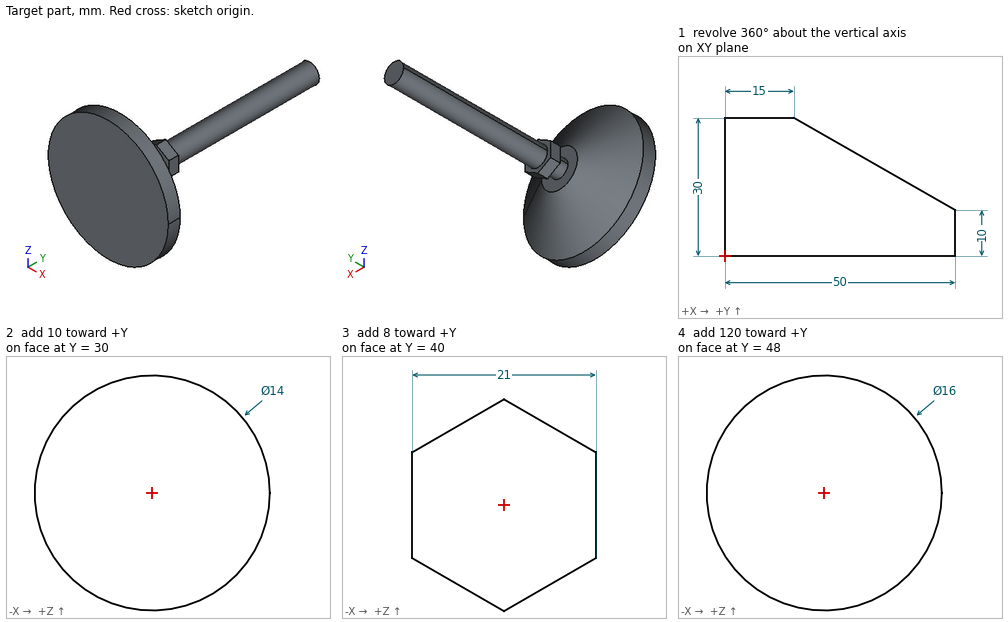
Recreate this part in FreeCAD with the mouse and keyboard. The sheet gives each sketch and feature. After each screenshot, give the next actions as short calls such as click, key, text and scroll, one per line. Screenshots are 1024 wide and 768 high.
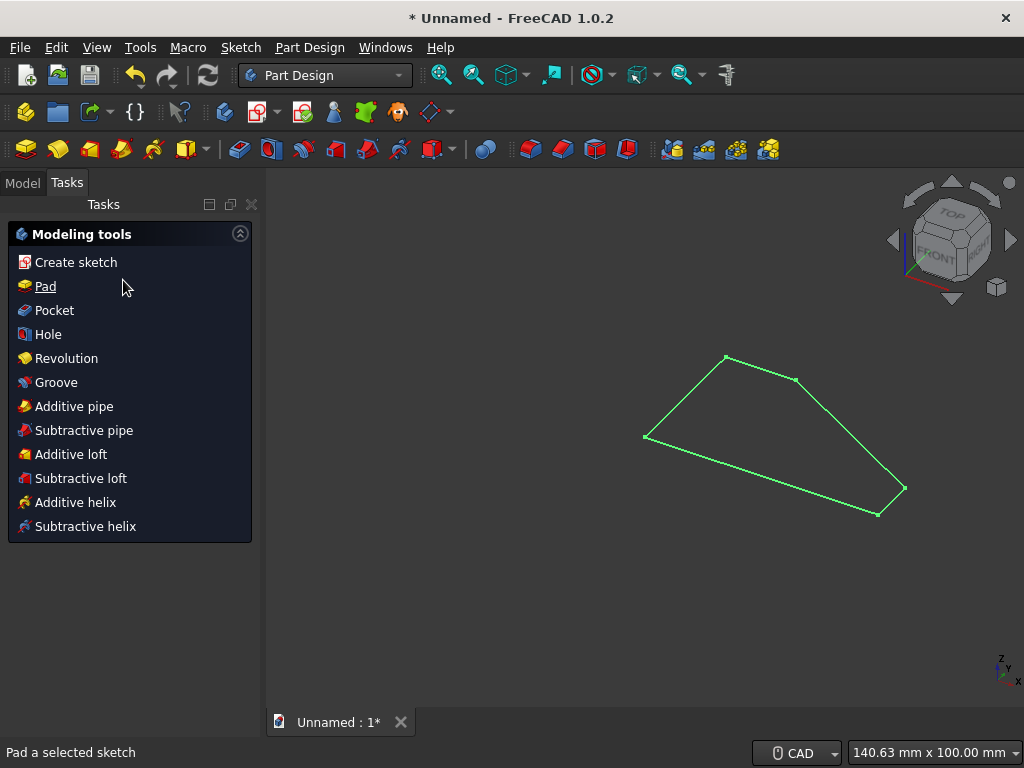
click(58, 150)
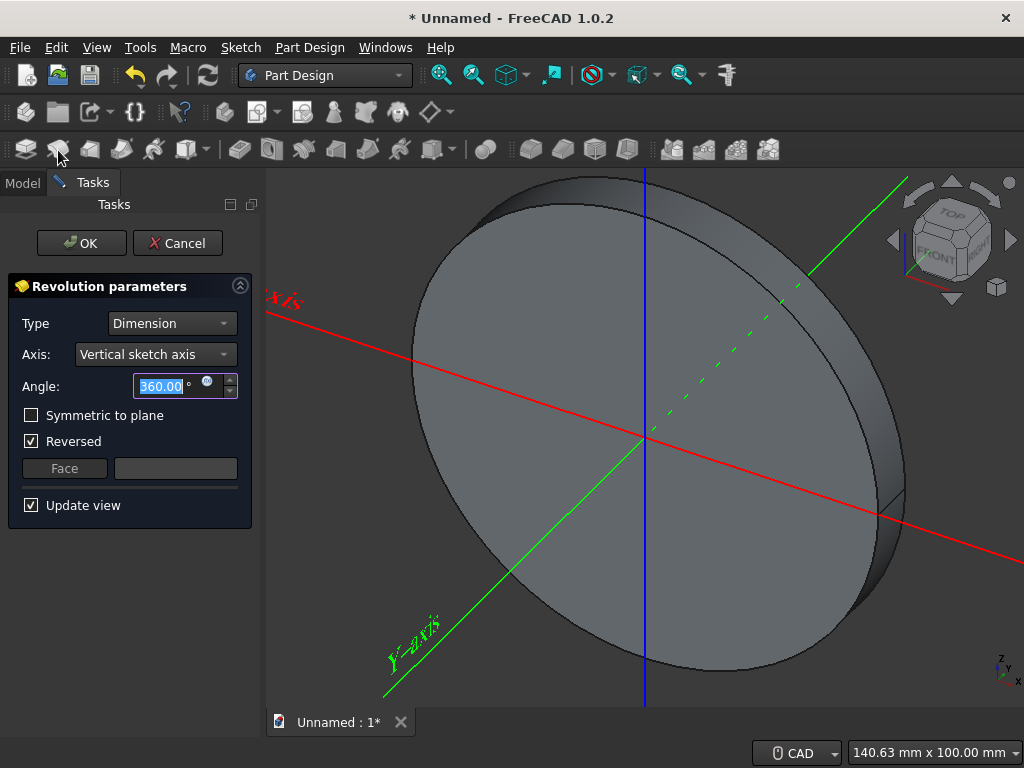
click(82, 243)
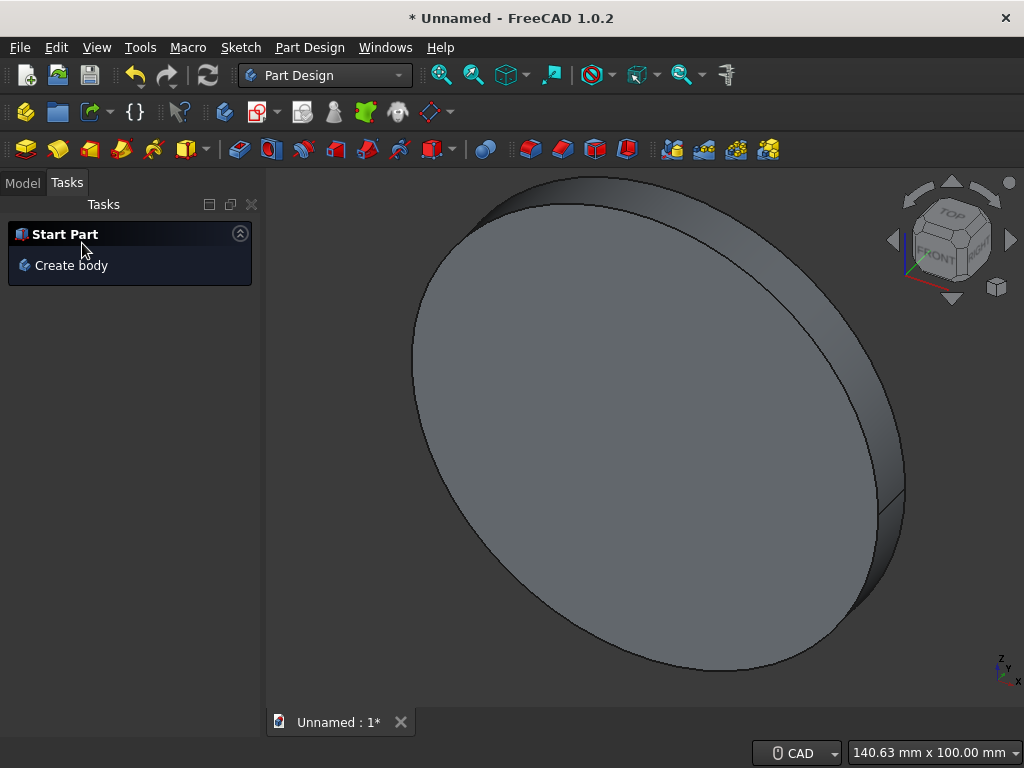
click(442, 76)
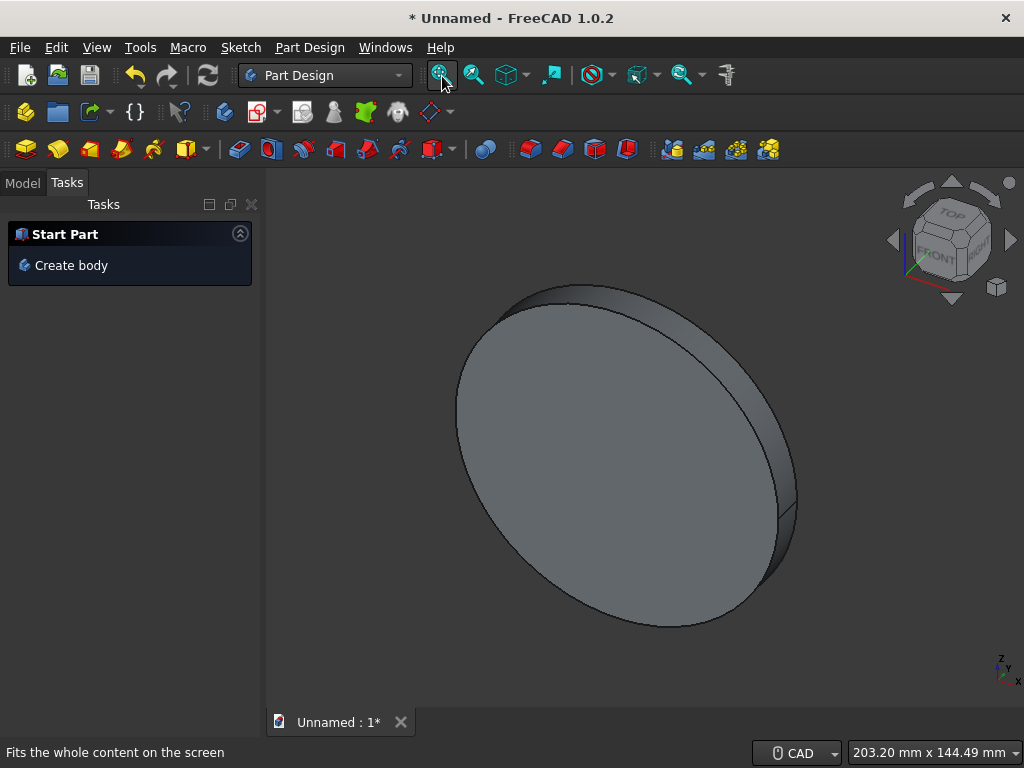
key(4)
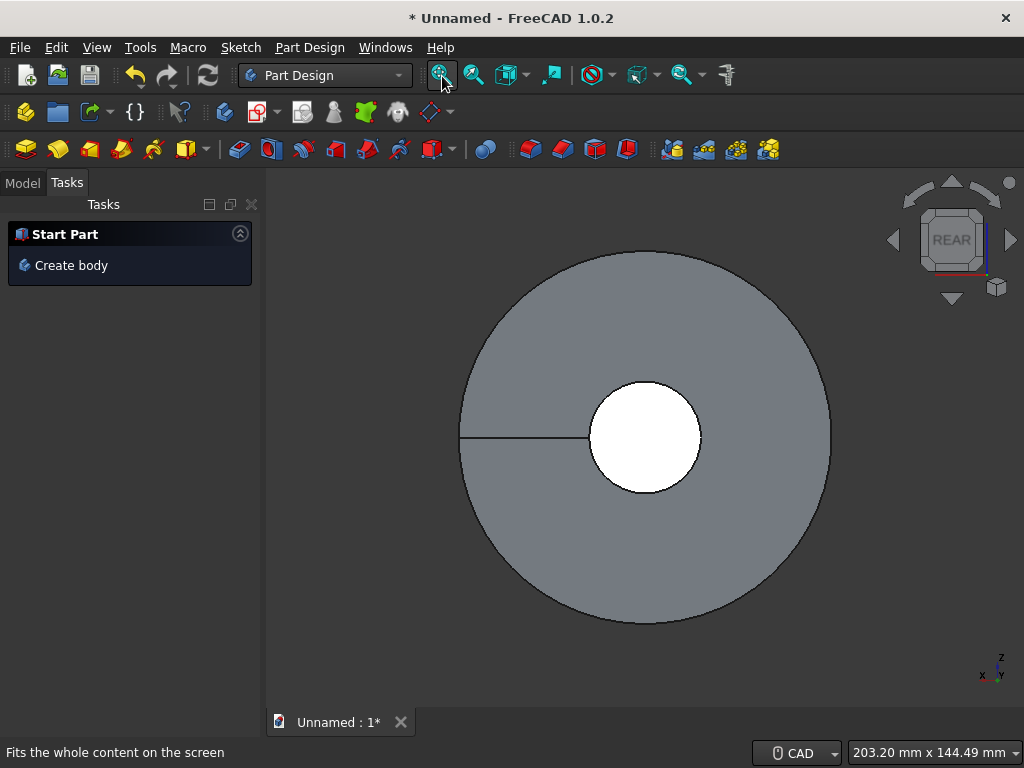
click(645, 436)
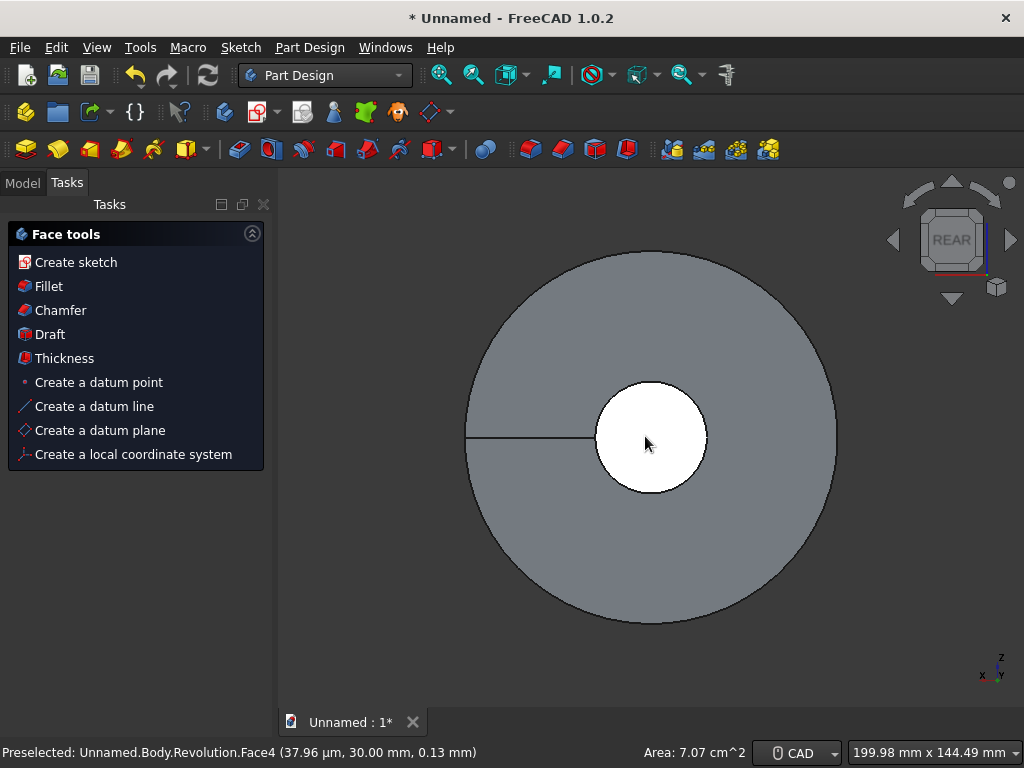
click(258, 112)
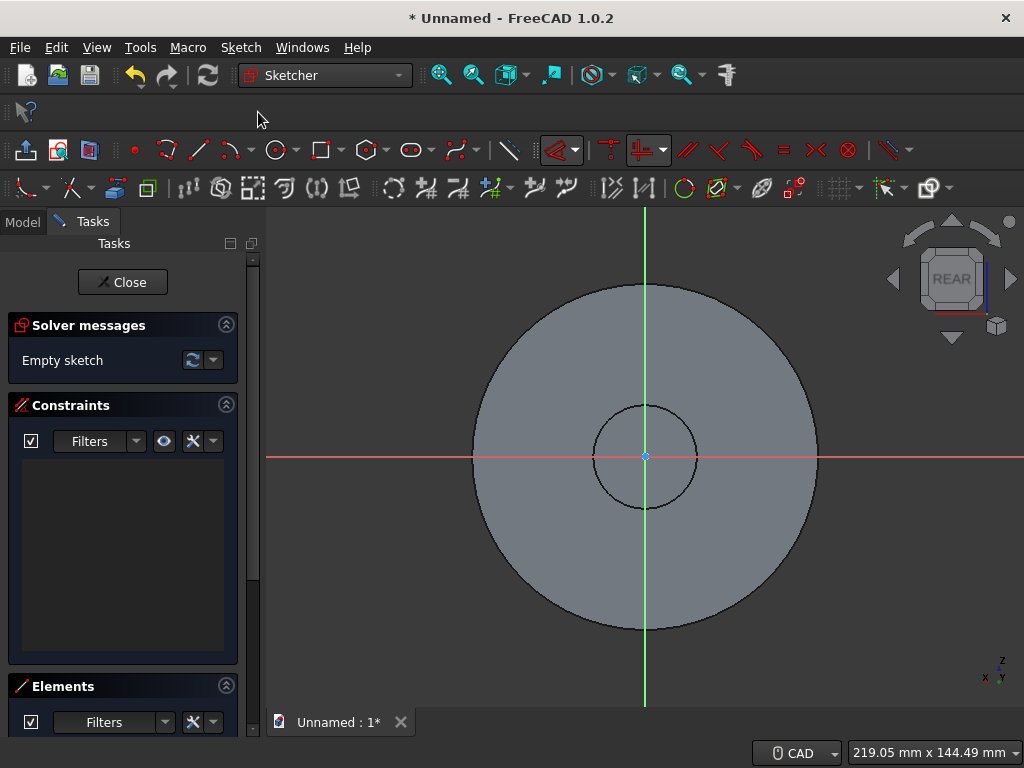
scroll(659, 457, up, 9)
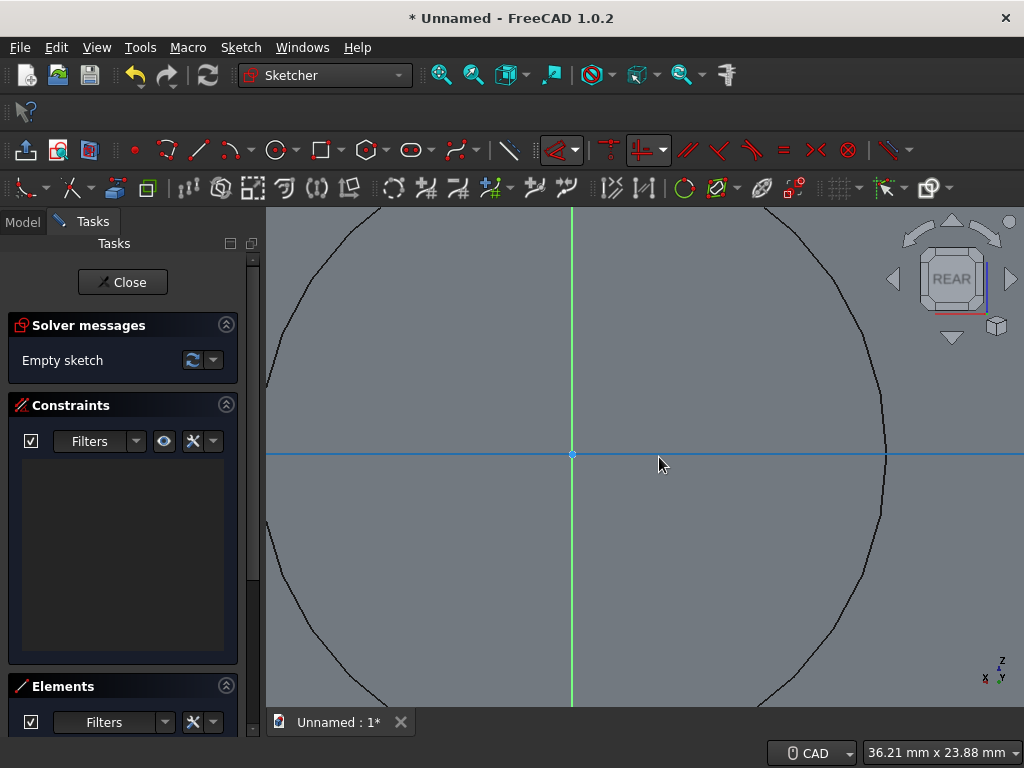
click(276, 150)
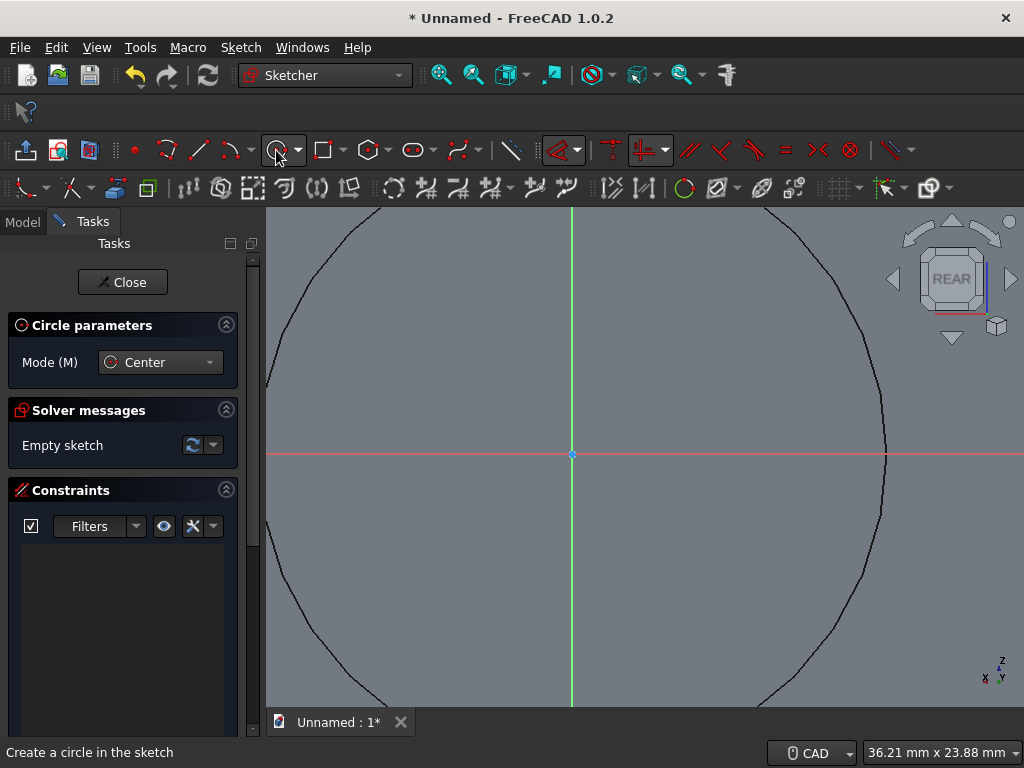
click(572, 454)
move(676, 351)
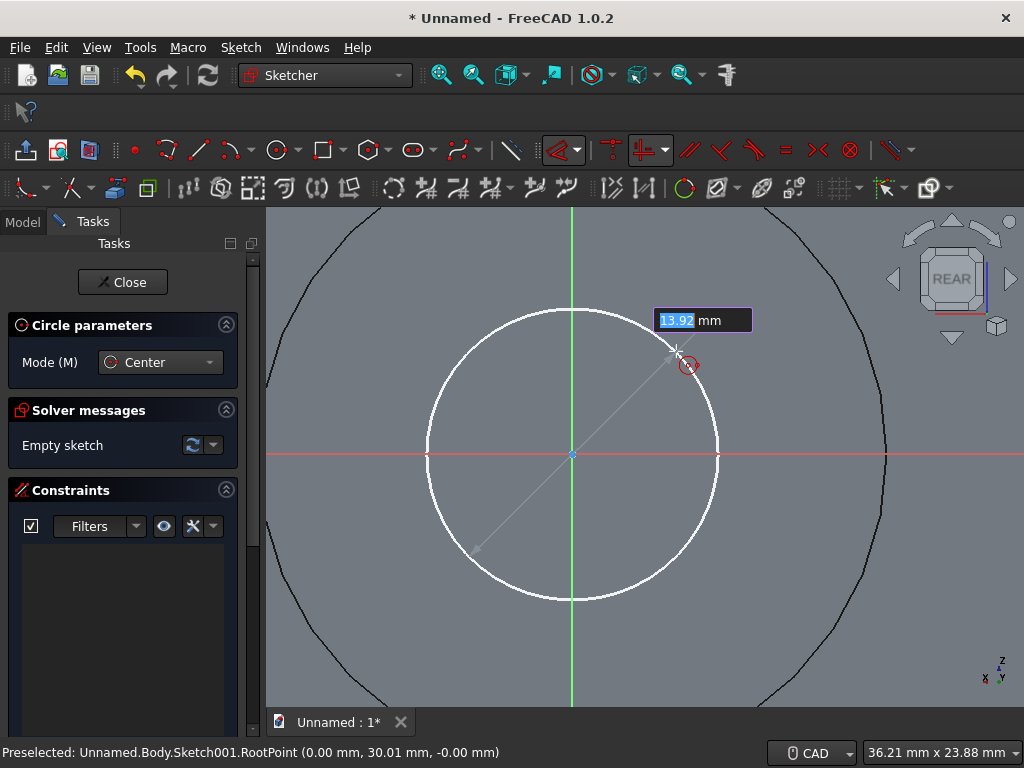
text(14)
key(Return)
key(Escape)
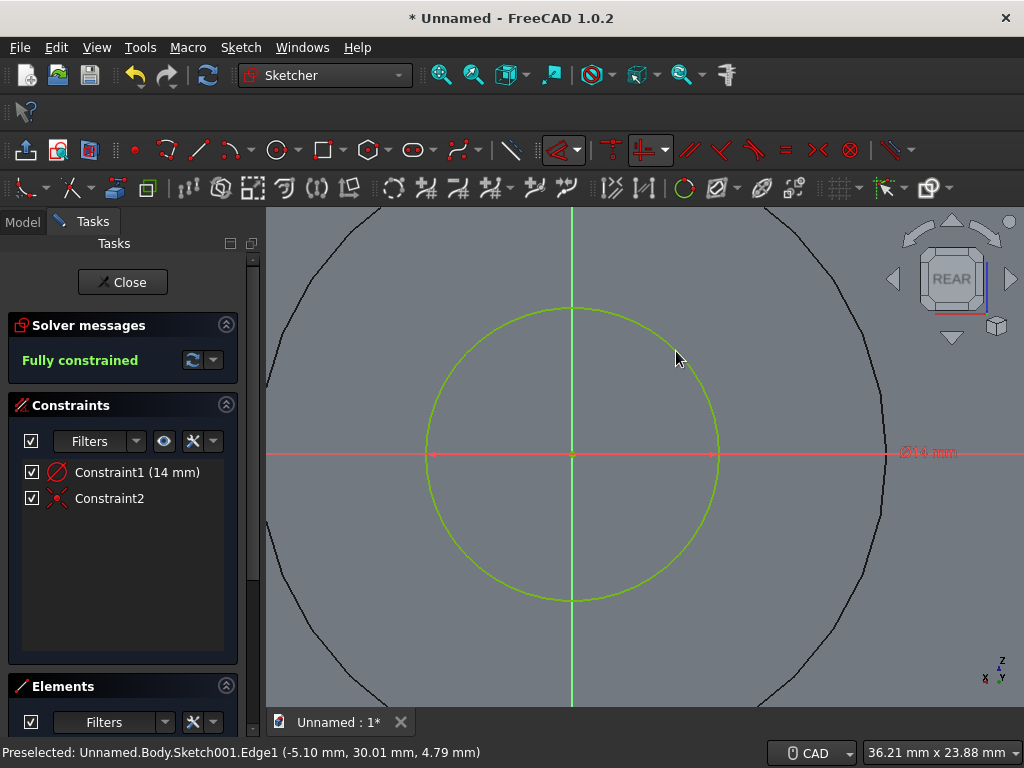
click(123, 282)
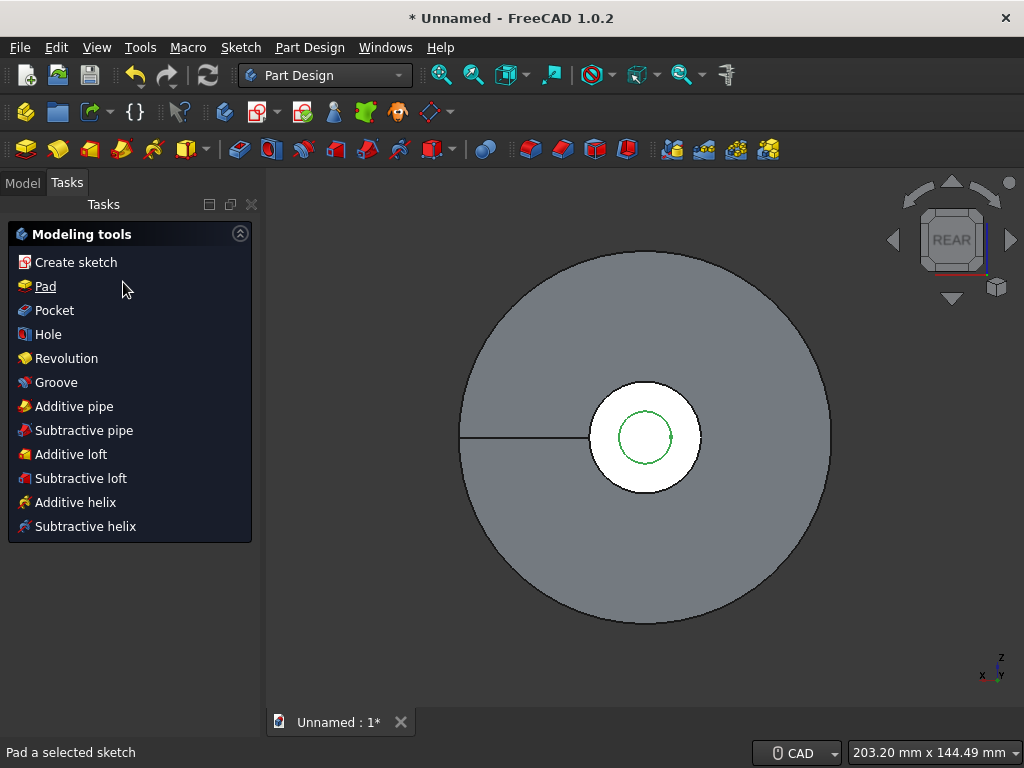
click(26, 150)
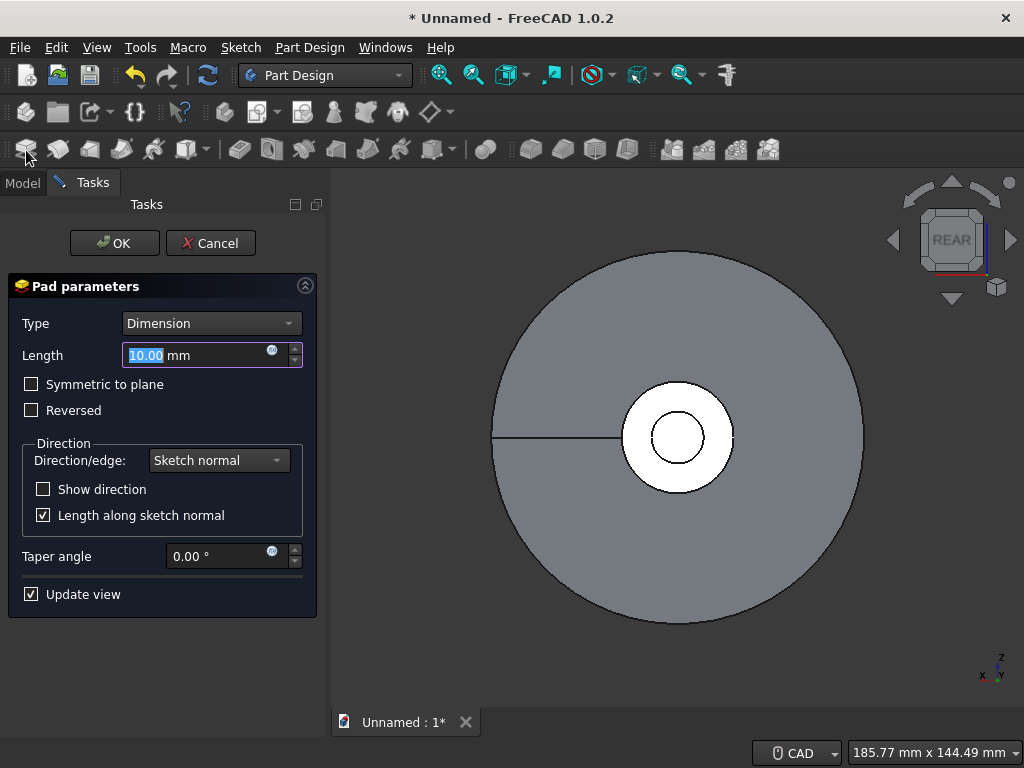
text(10)
key(Tab)